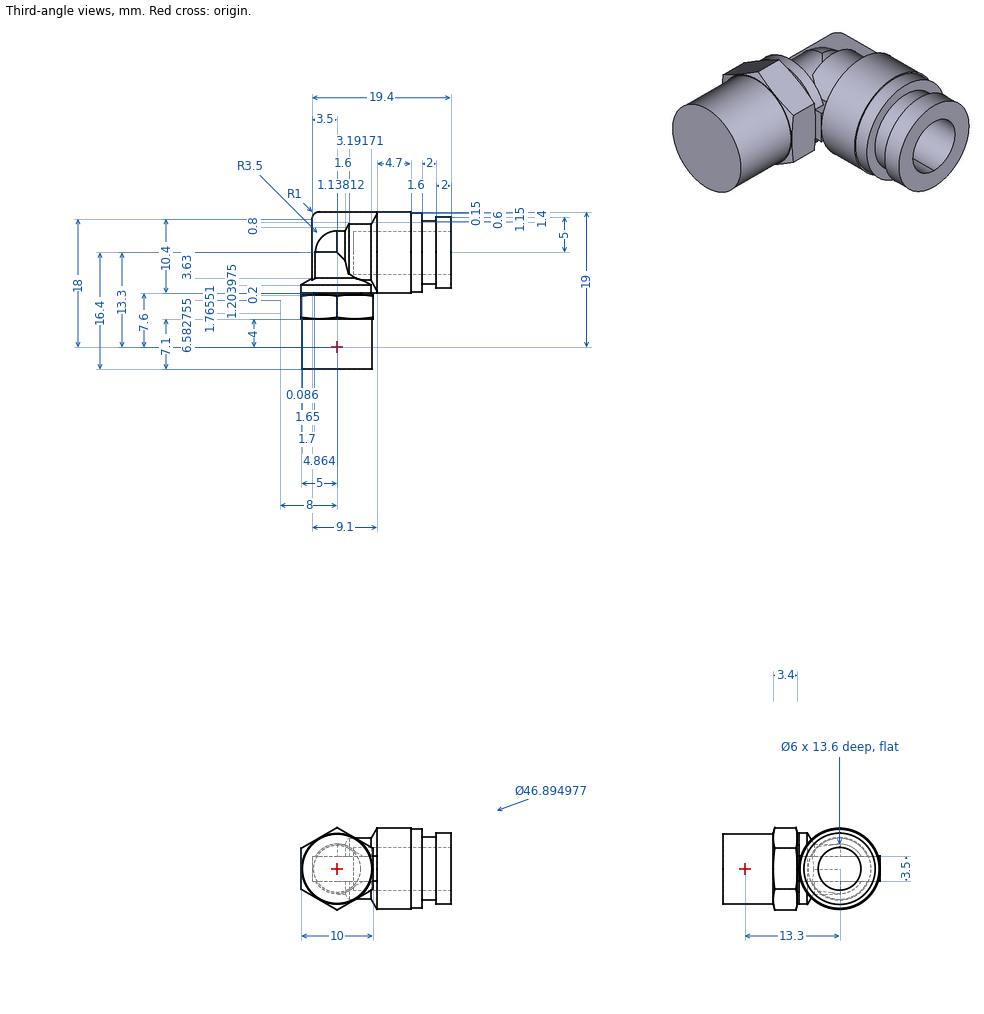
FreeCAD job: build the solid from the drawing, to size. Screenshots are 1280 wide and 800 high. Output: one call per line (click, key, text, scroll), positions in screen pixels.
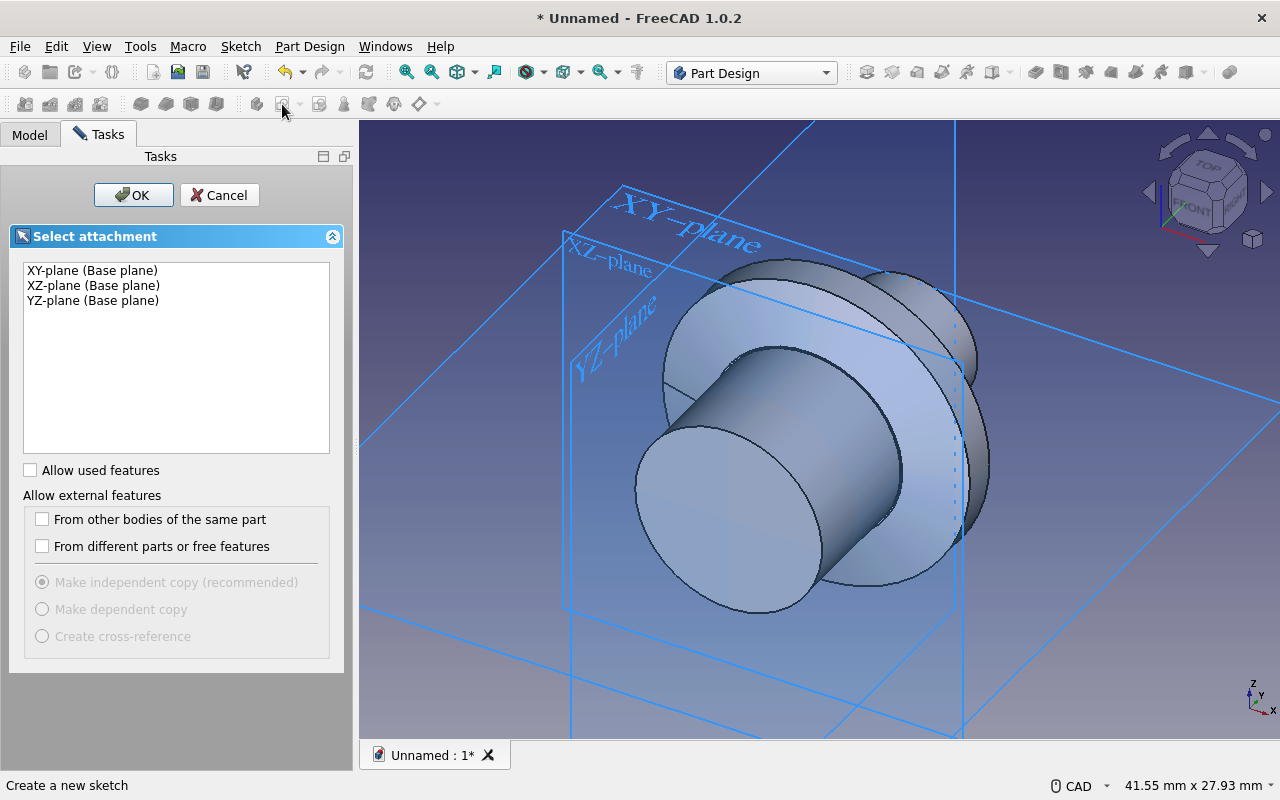
click(84, 270)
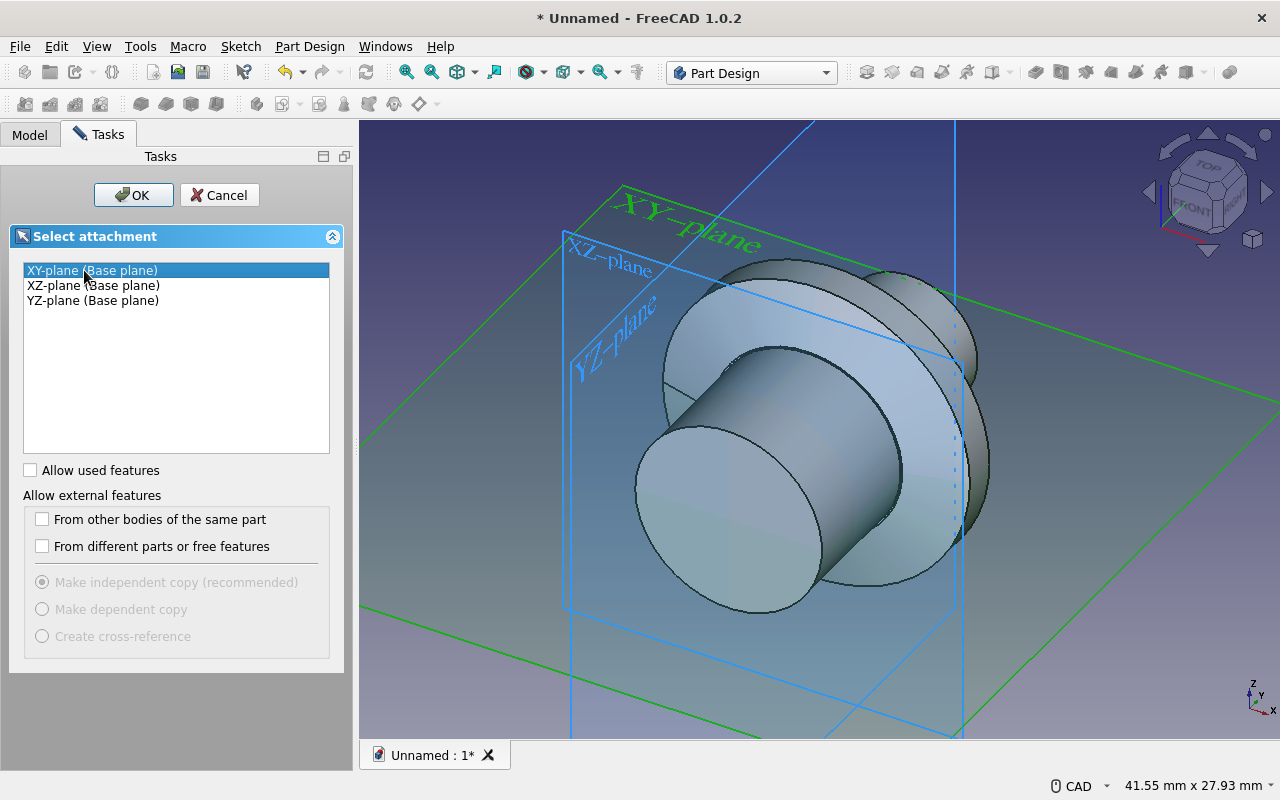
click(134, 195)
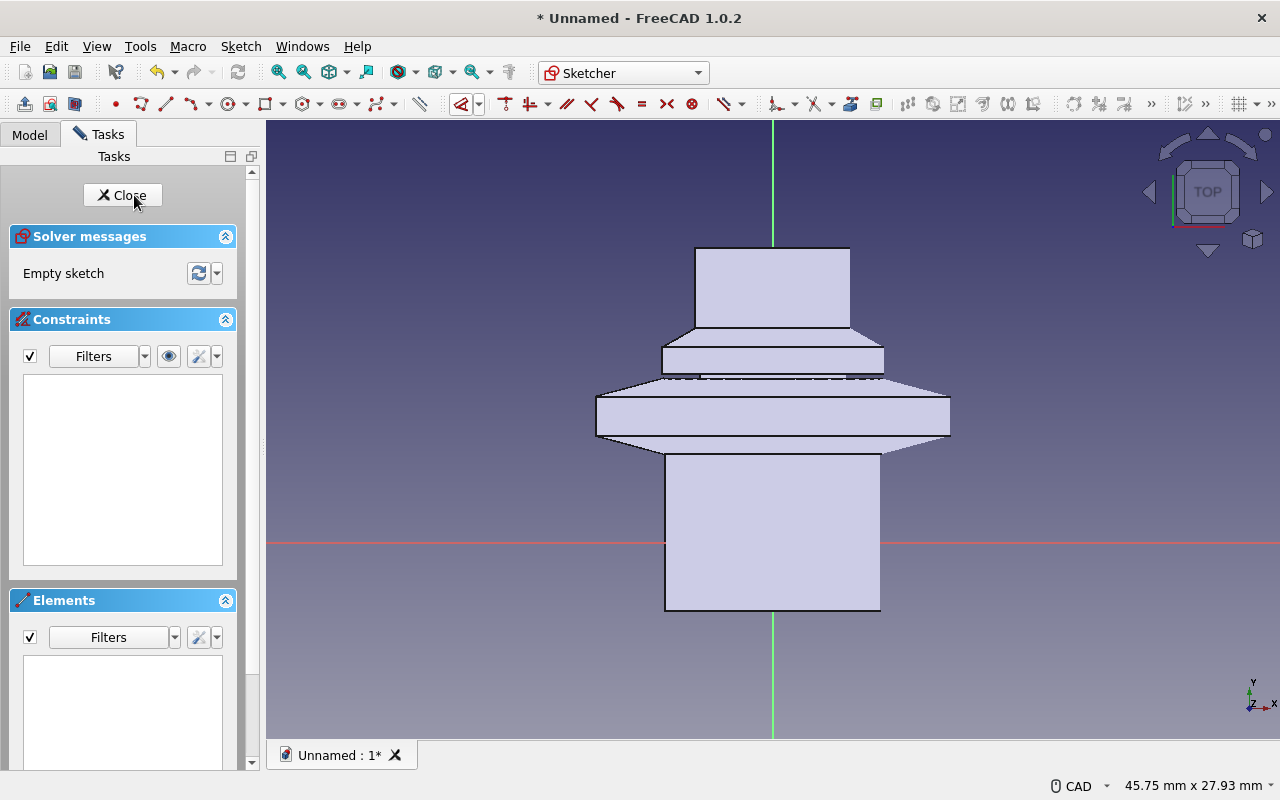
key(q)
key(s)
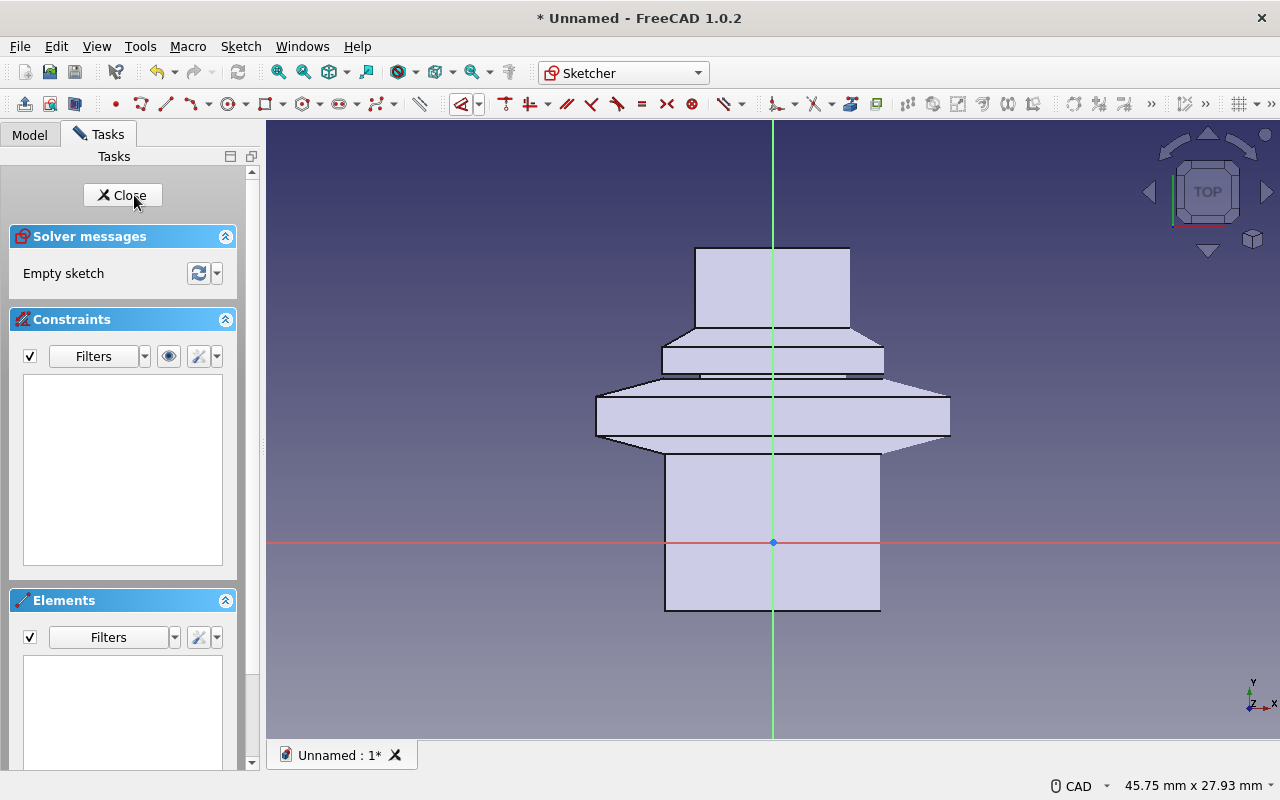
scroll(294, 711, down, 1)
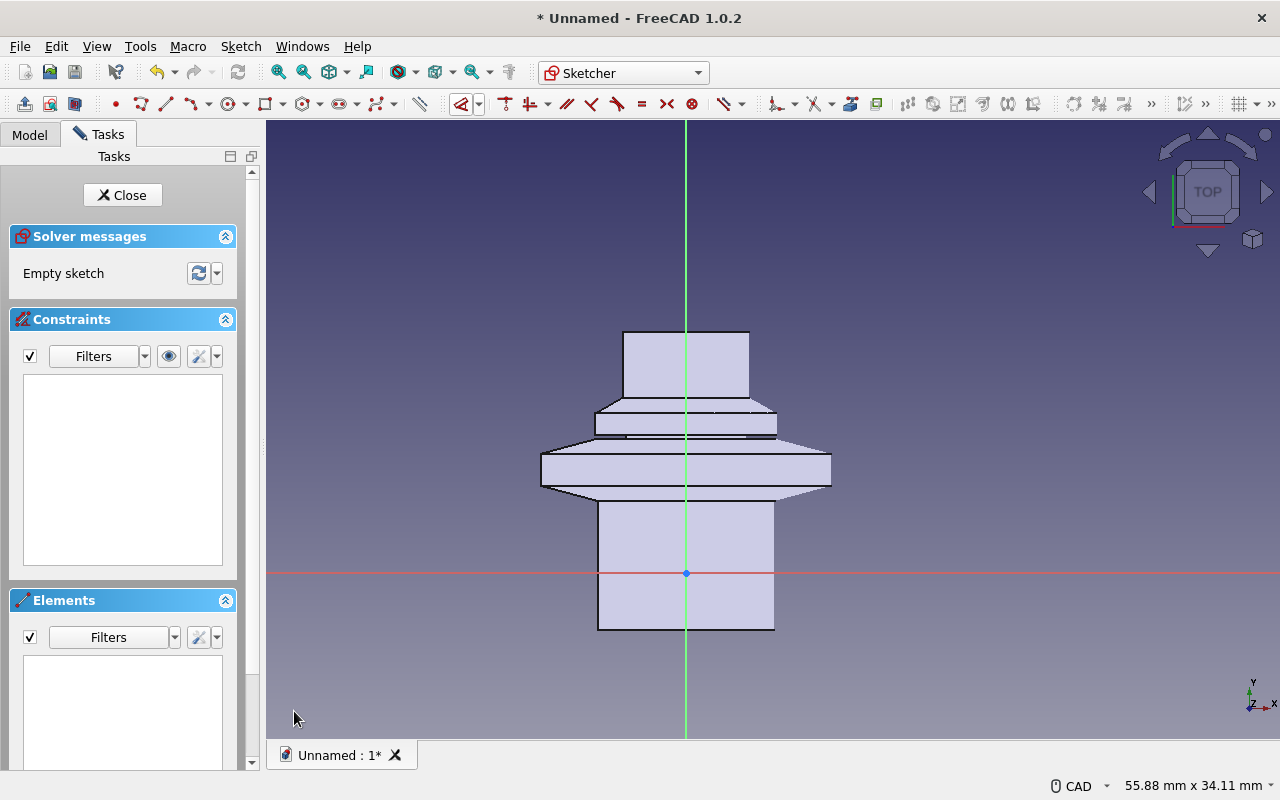
key(g)
key(m)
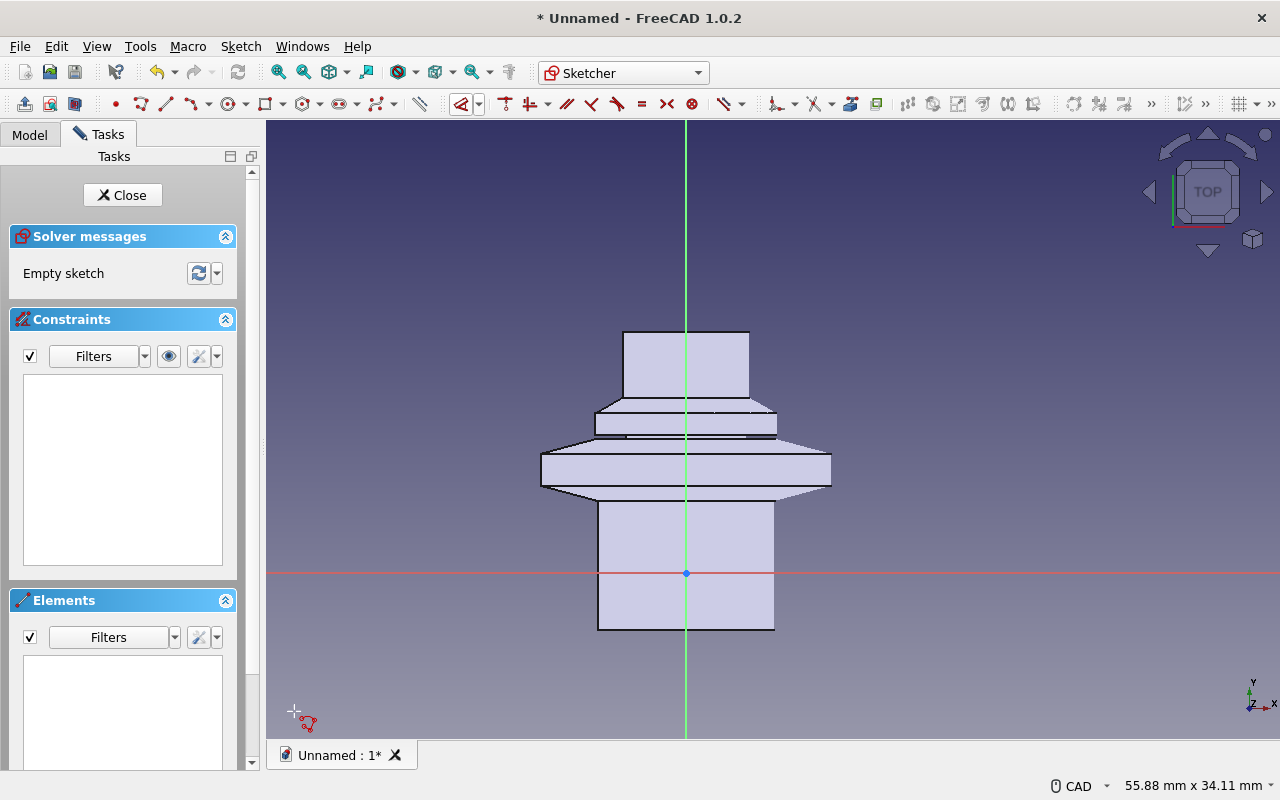
click(623, 247)
click(623, 435)
click(788, 435)
click(788, 228)
click(641, 228)
right_click(641, 228)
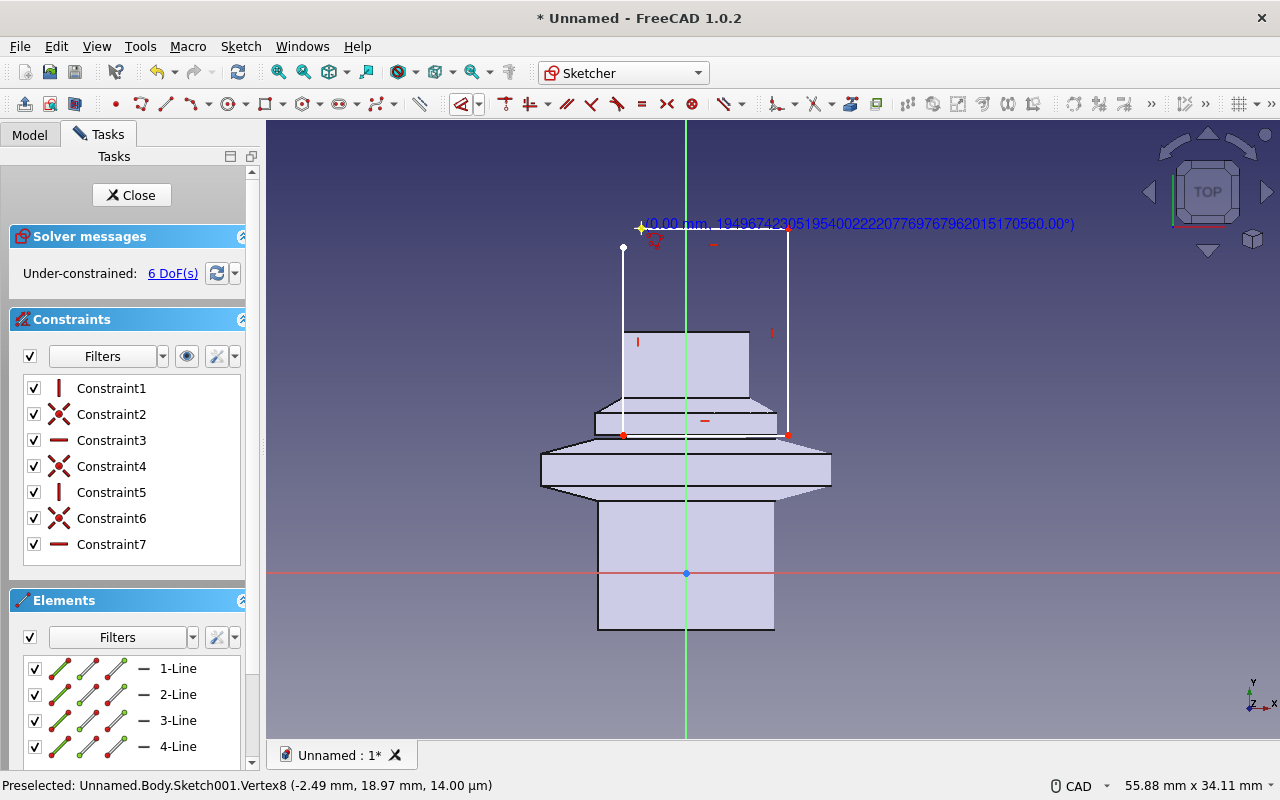
key(g)
key(3)
key(a)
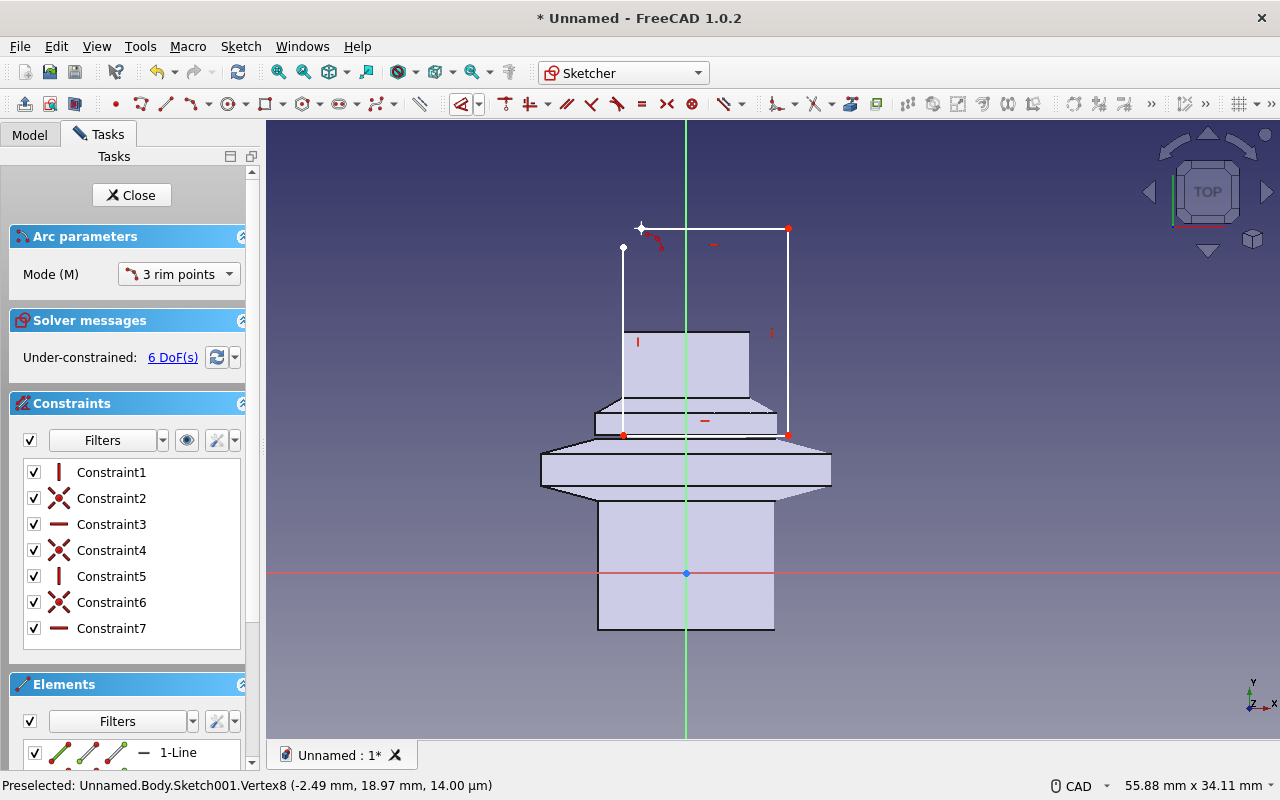
click(641, 229)
click(623, 248)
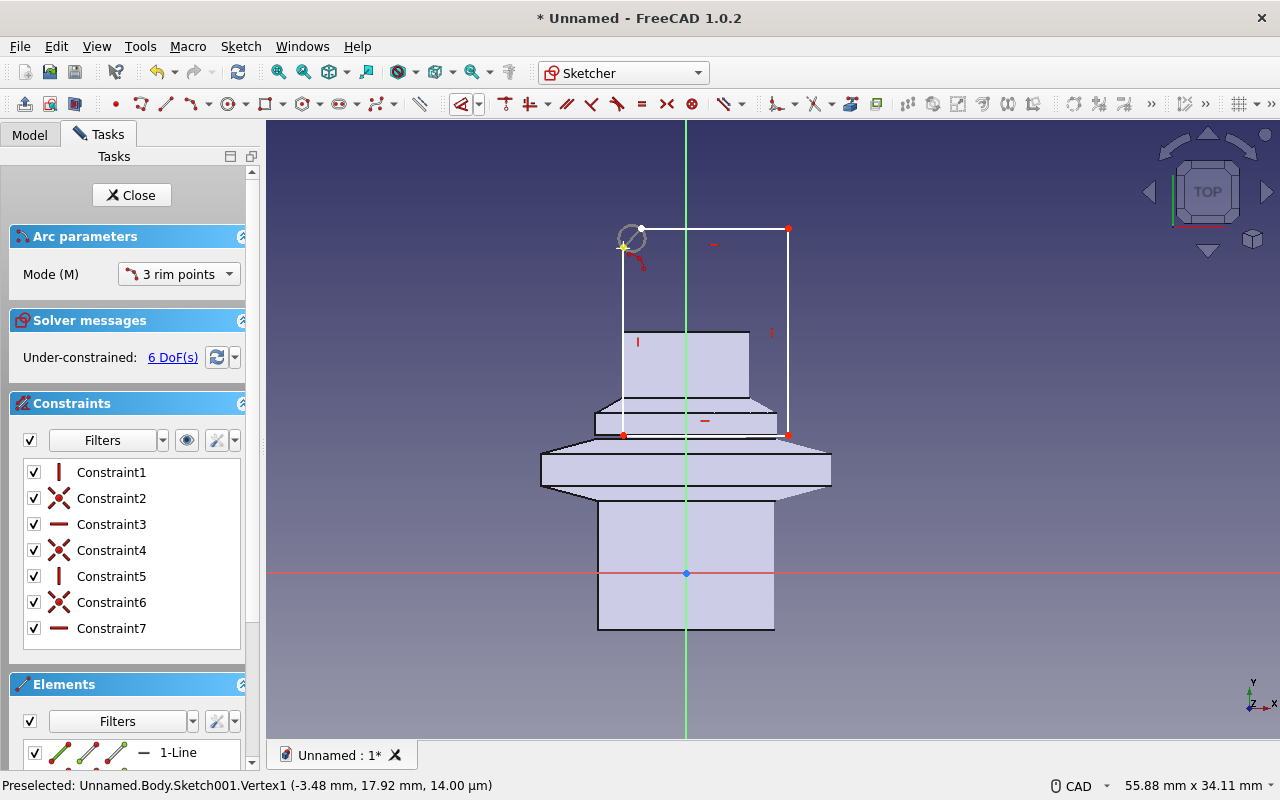
scroll(628, 234, up, 6)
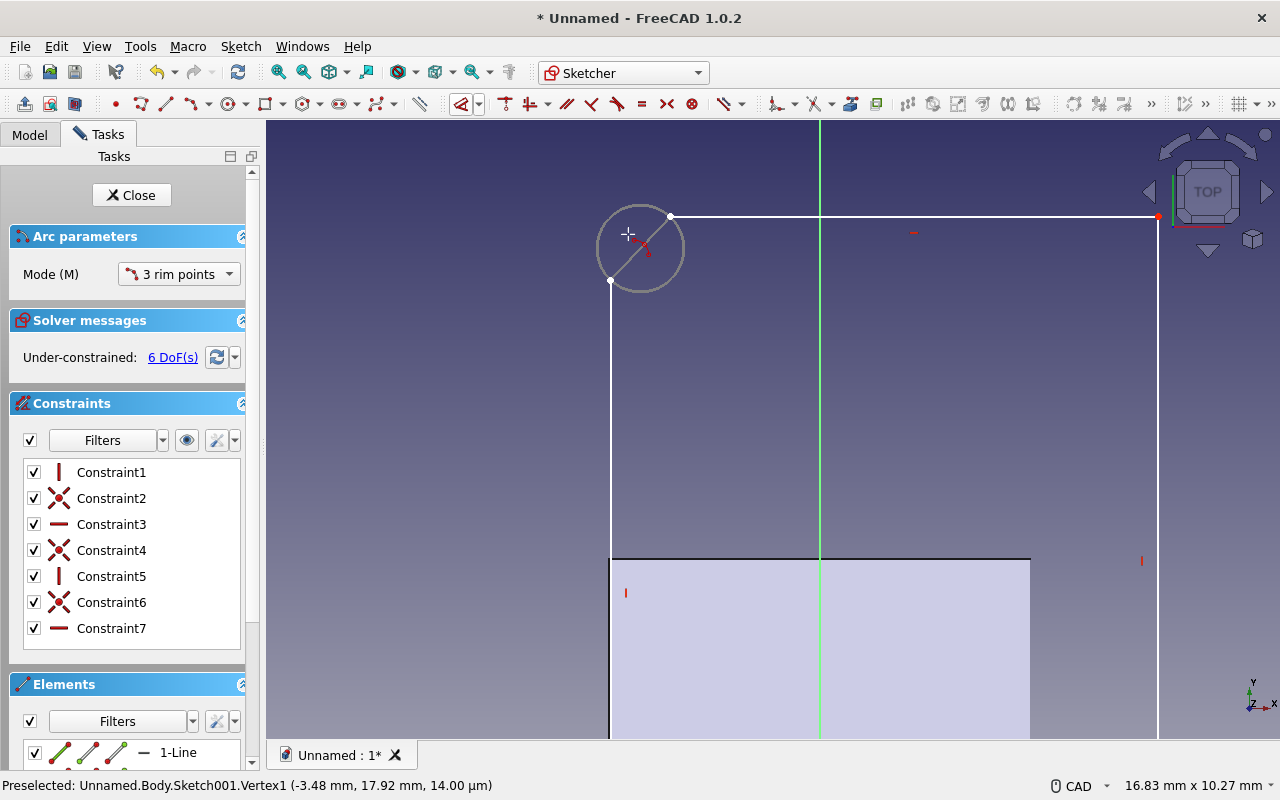
click(627, 233)
key(Escape)